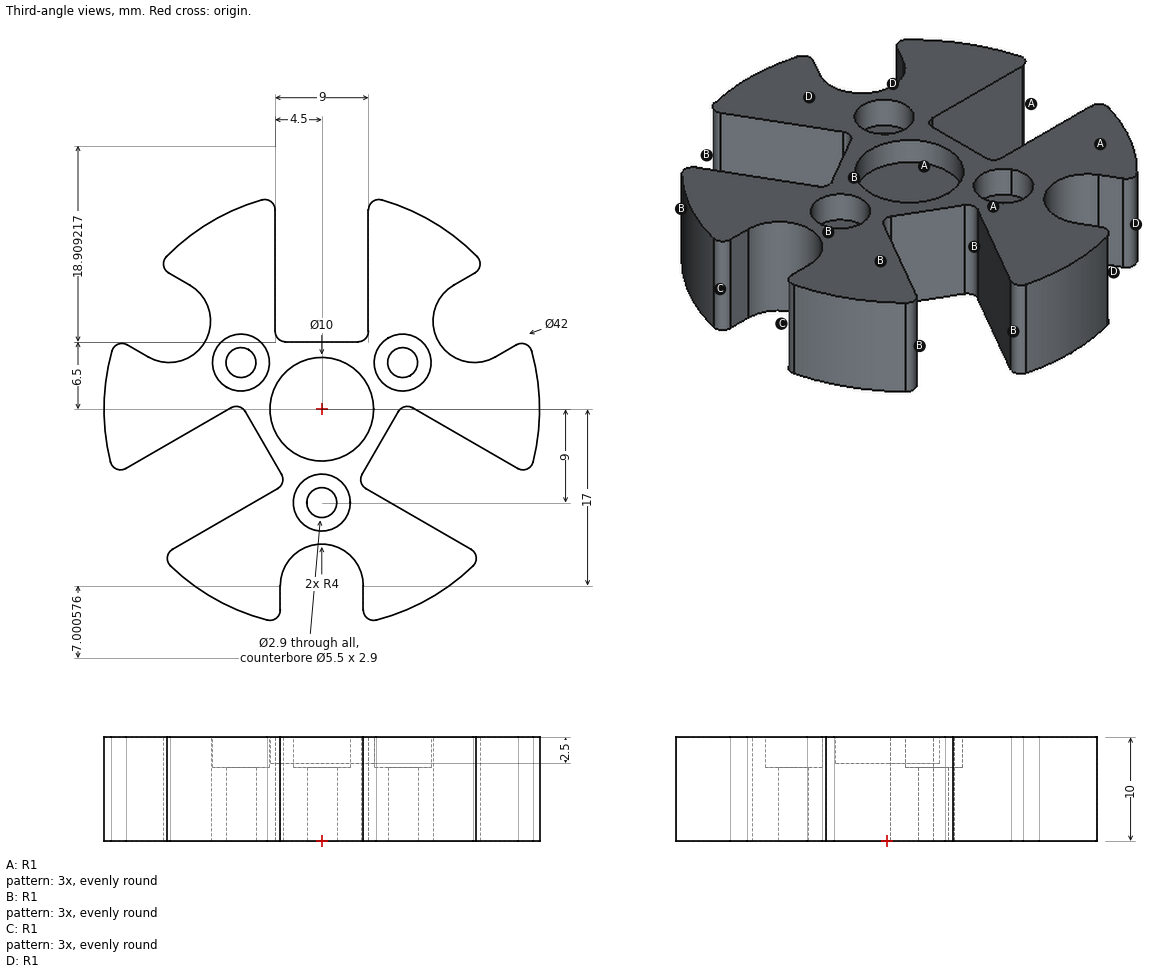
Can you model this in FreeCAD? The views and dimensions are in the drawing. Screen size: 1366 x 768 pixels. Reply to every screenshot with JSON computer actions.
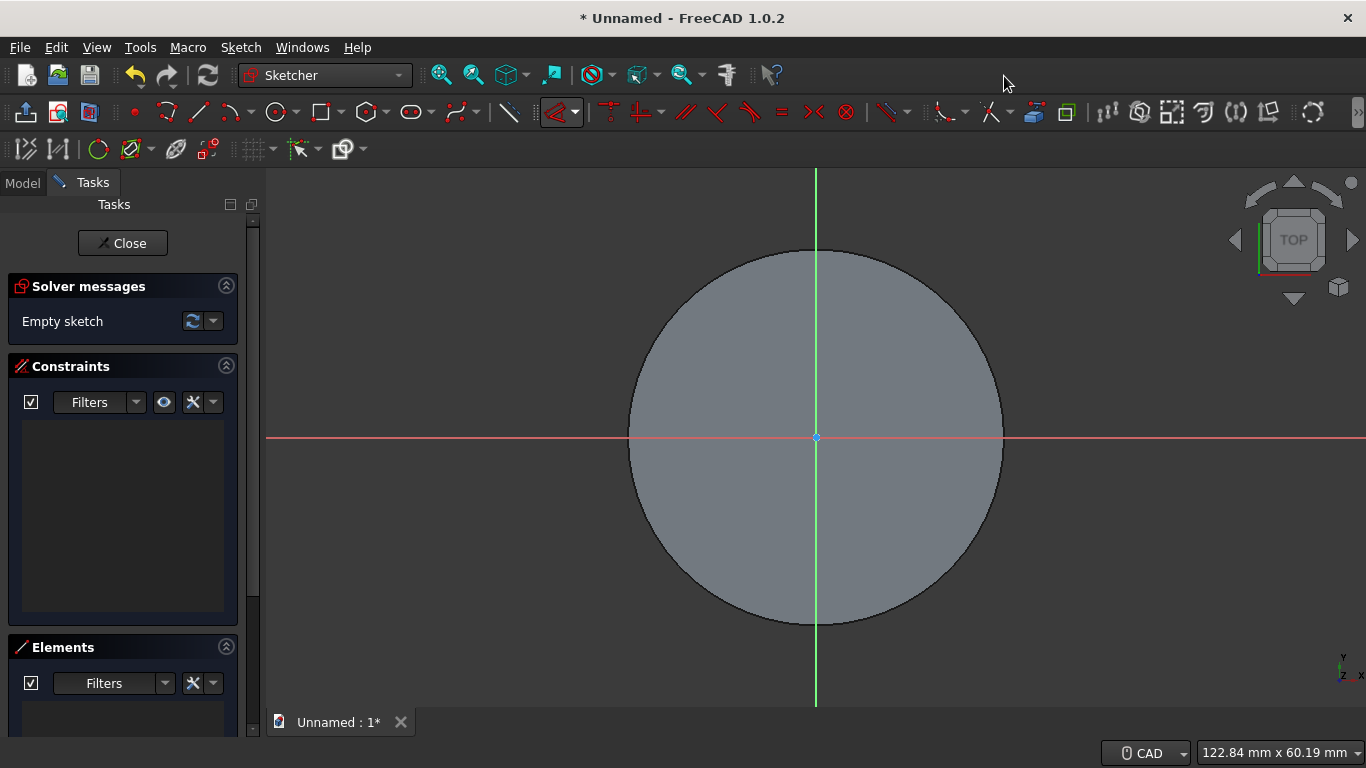
{"action": "scroll", "coordinate": [438, 679], "scroll_direction": "down", "scroll_amount": 1}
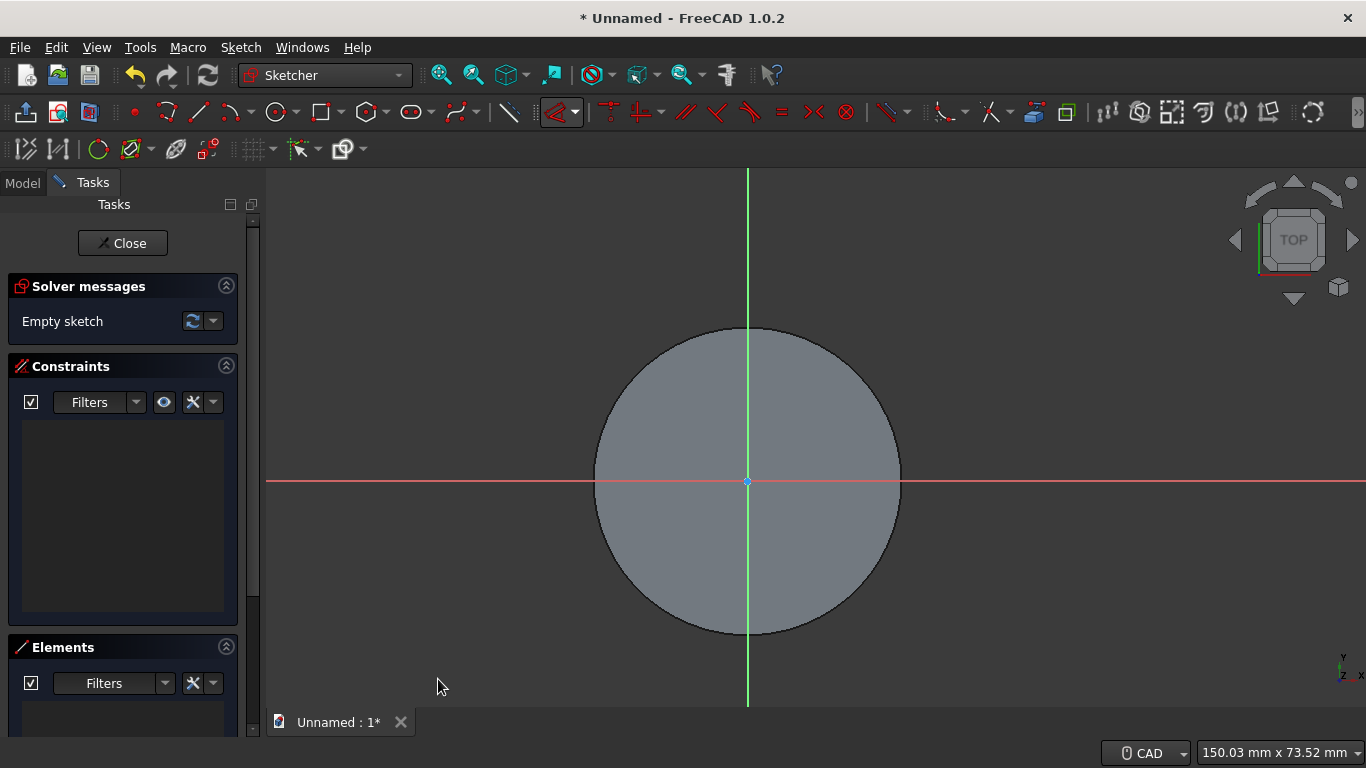
{"action": "scroll", "coordinate": [748, 328], "scroll_direction": "up", "scroll_amount": 3}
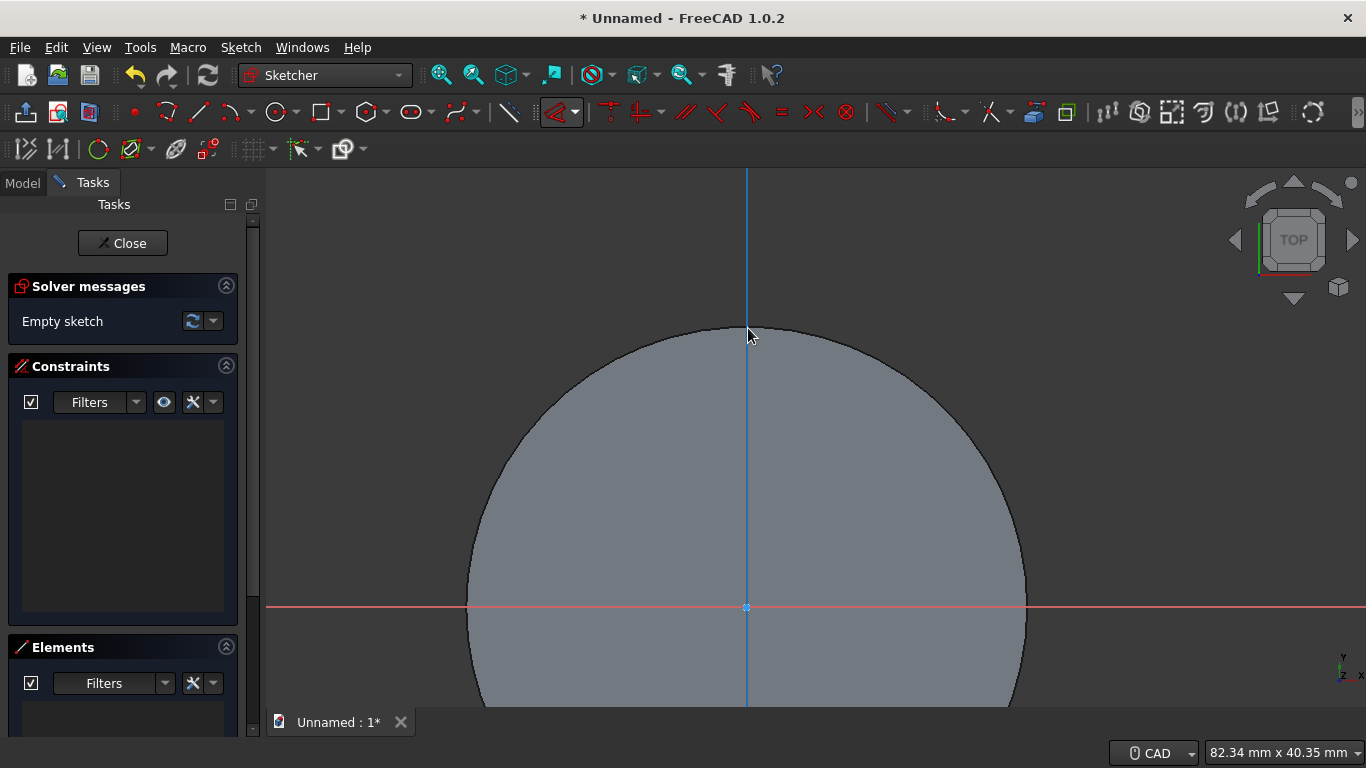
{"action": "left_click", "coordinate": [322, 112]}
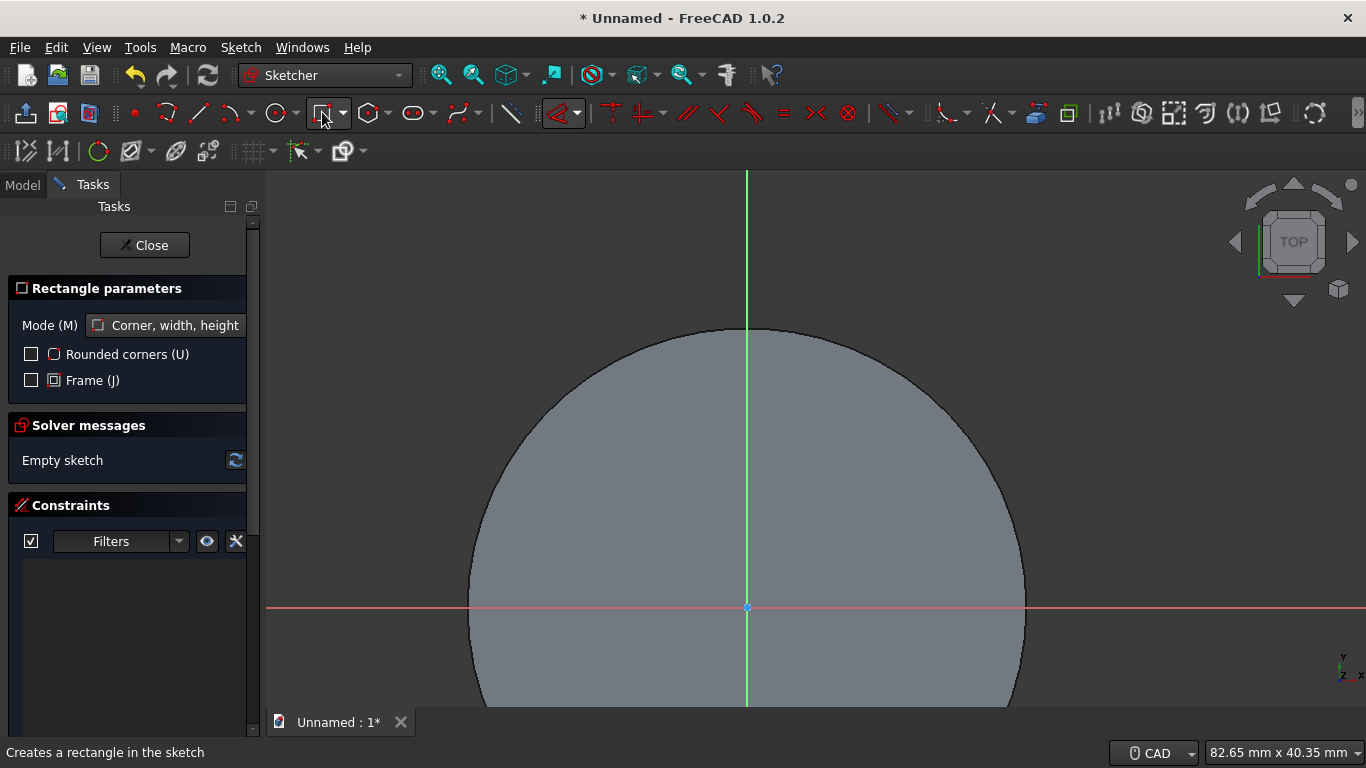
{"action": "left_click", "coordinate": [687, 270]}
{"action": "left_click", "coordinate": [807, 521]}
{"action": "key", "text": "Escape"}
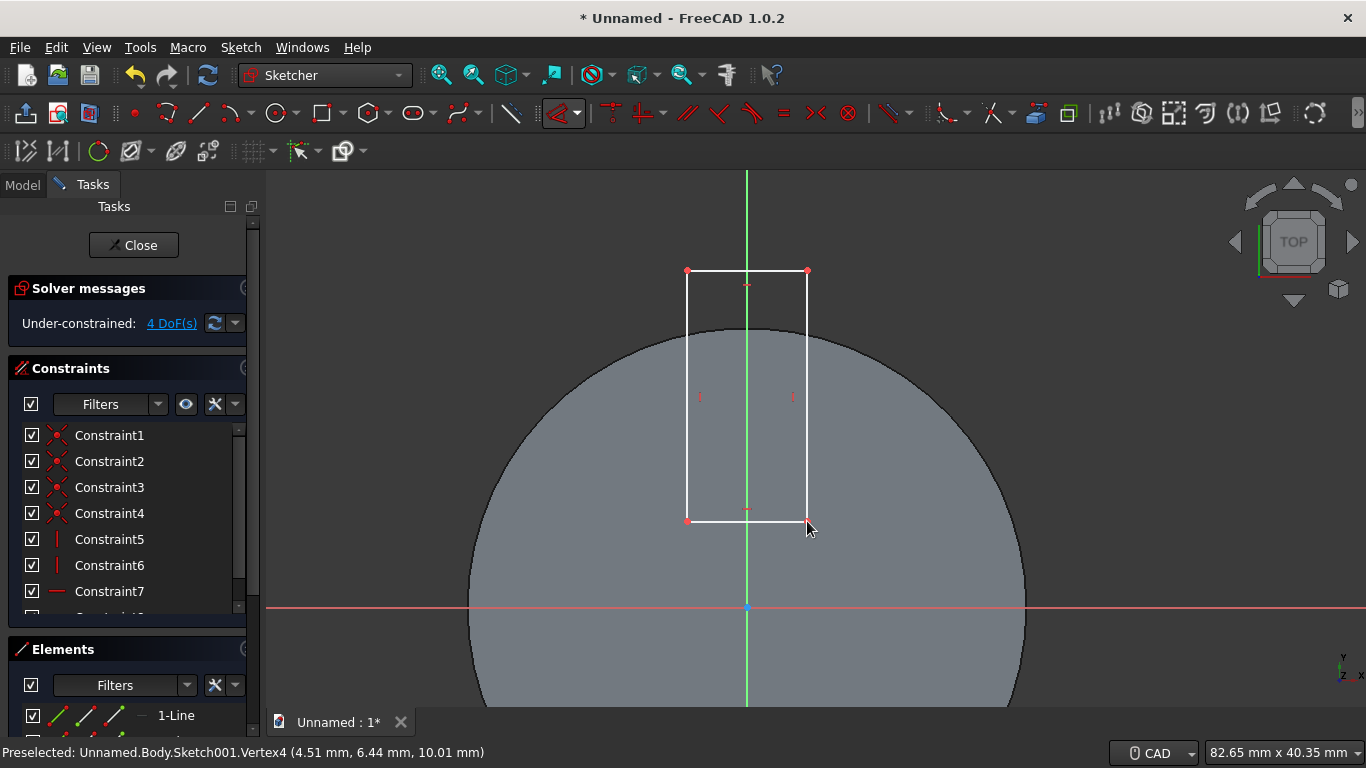
{"action": "left_click", "coordinate": [723, 522]}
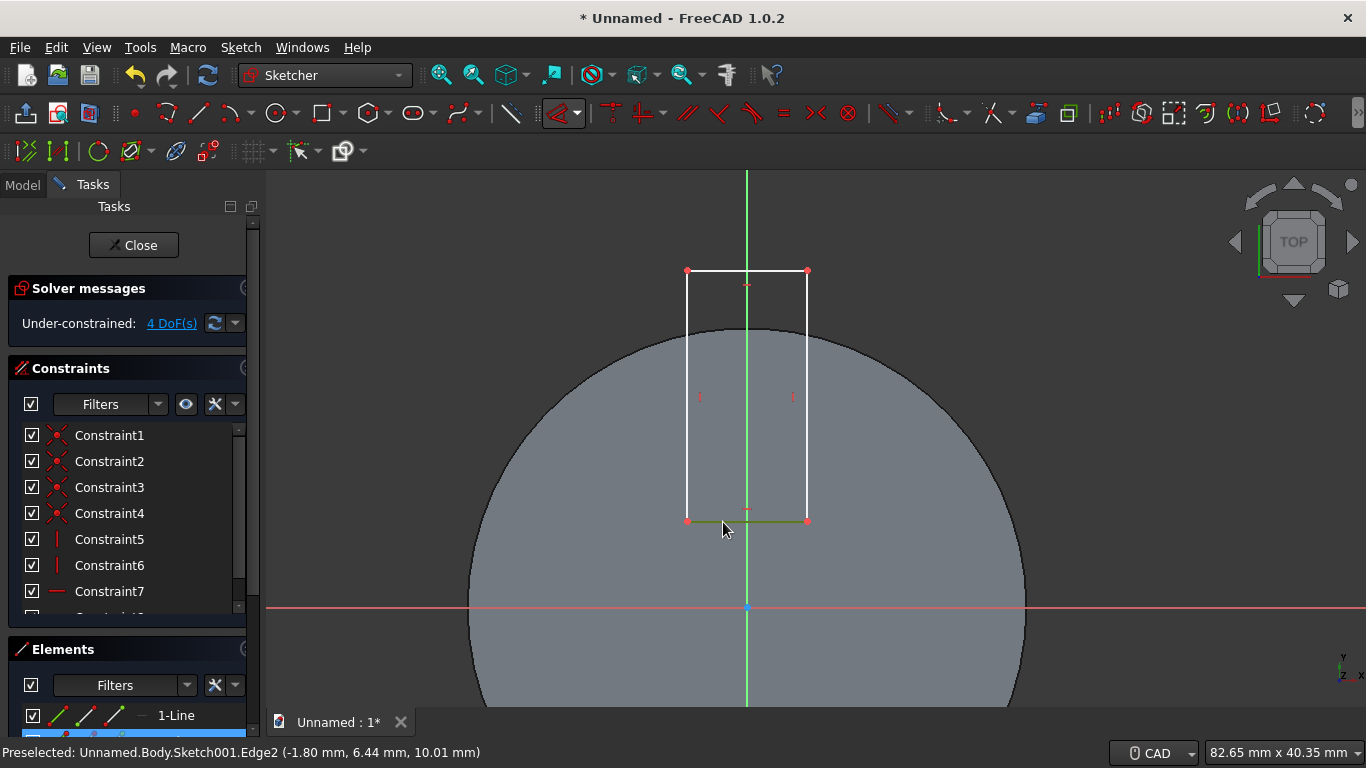
{"action": "key", "text": "l"}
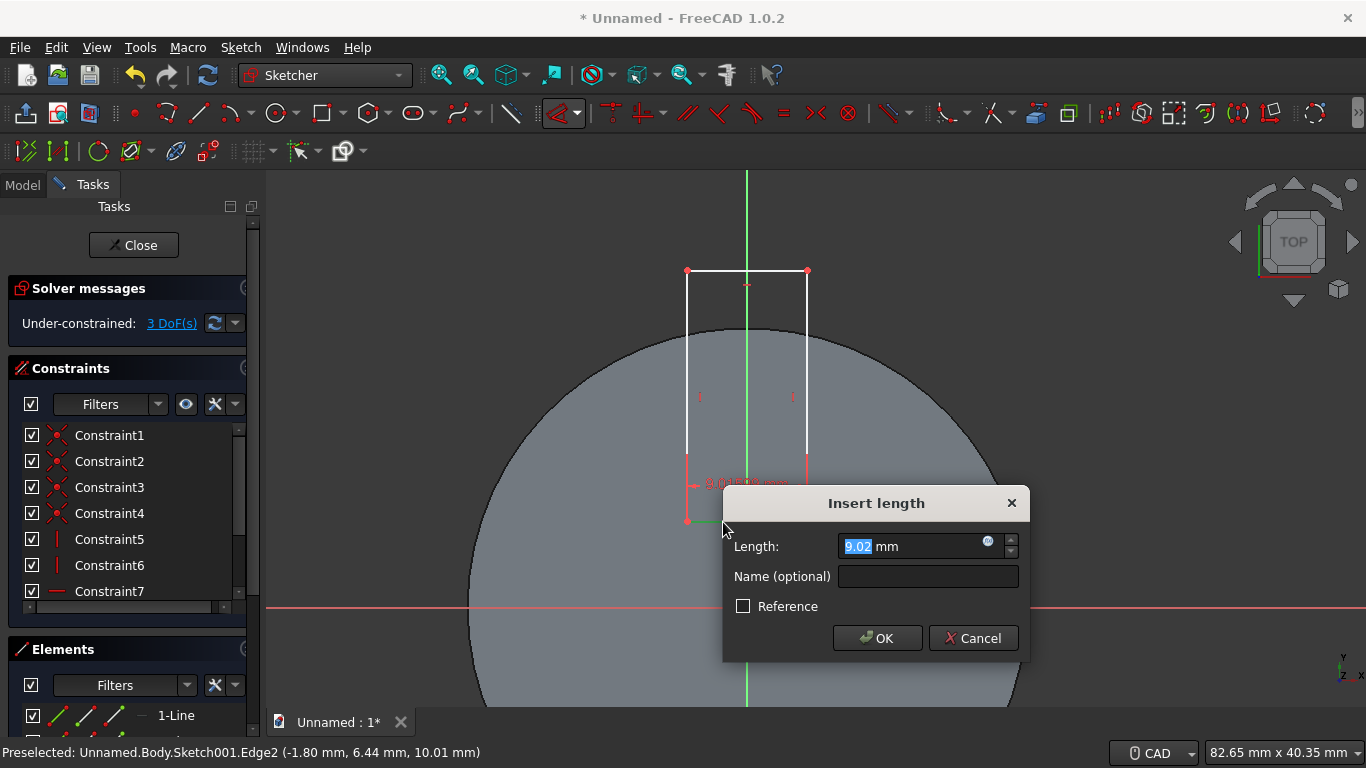
{"action": "type", "text": "9"}
{"action": "key", "text": "Return"}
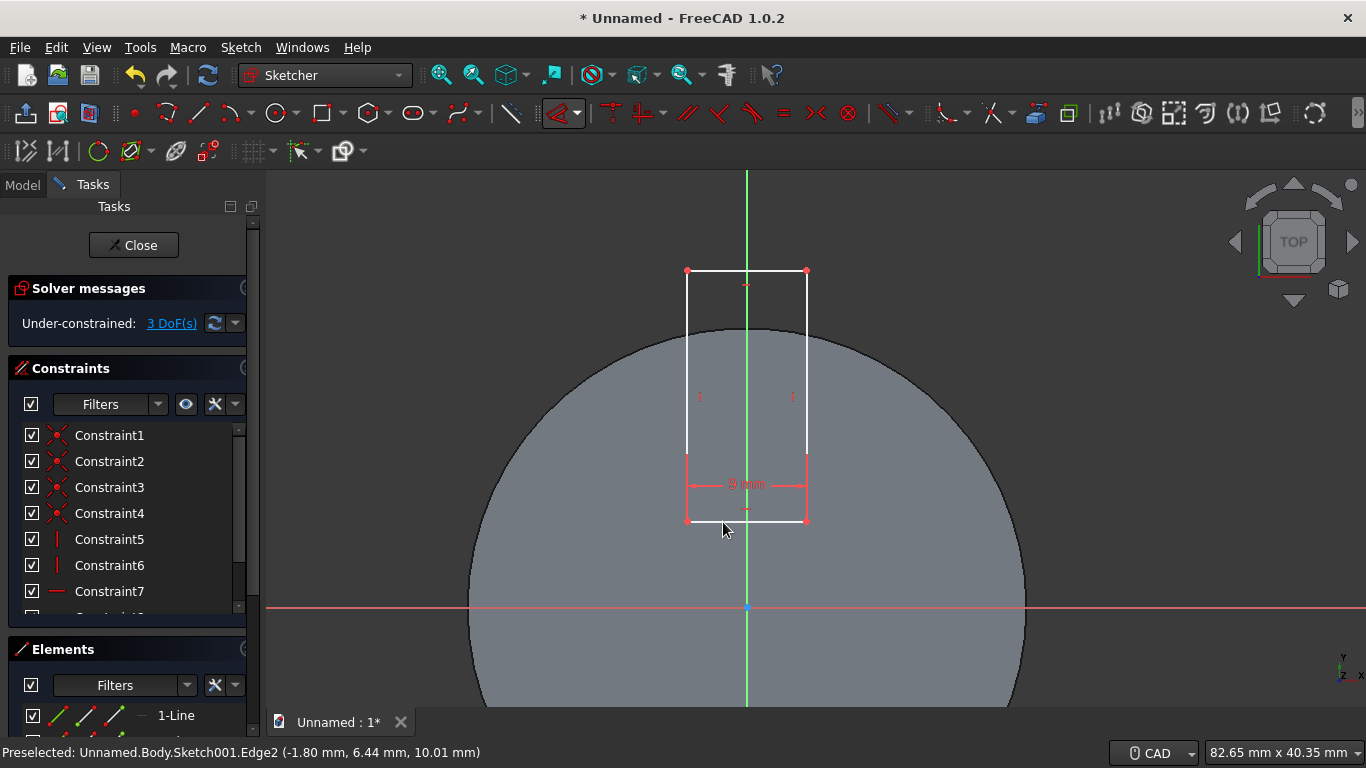
{"action": "left_click", "coordinate": [687, 271]}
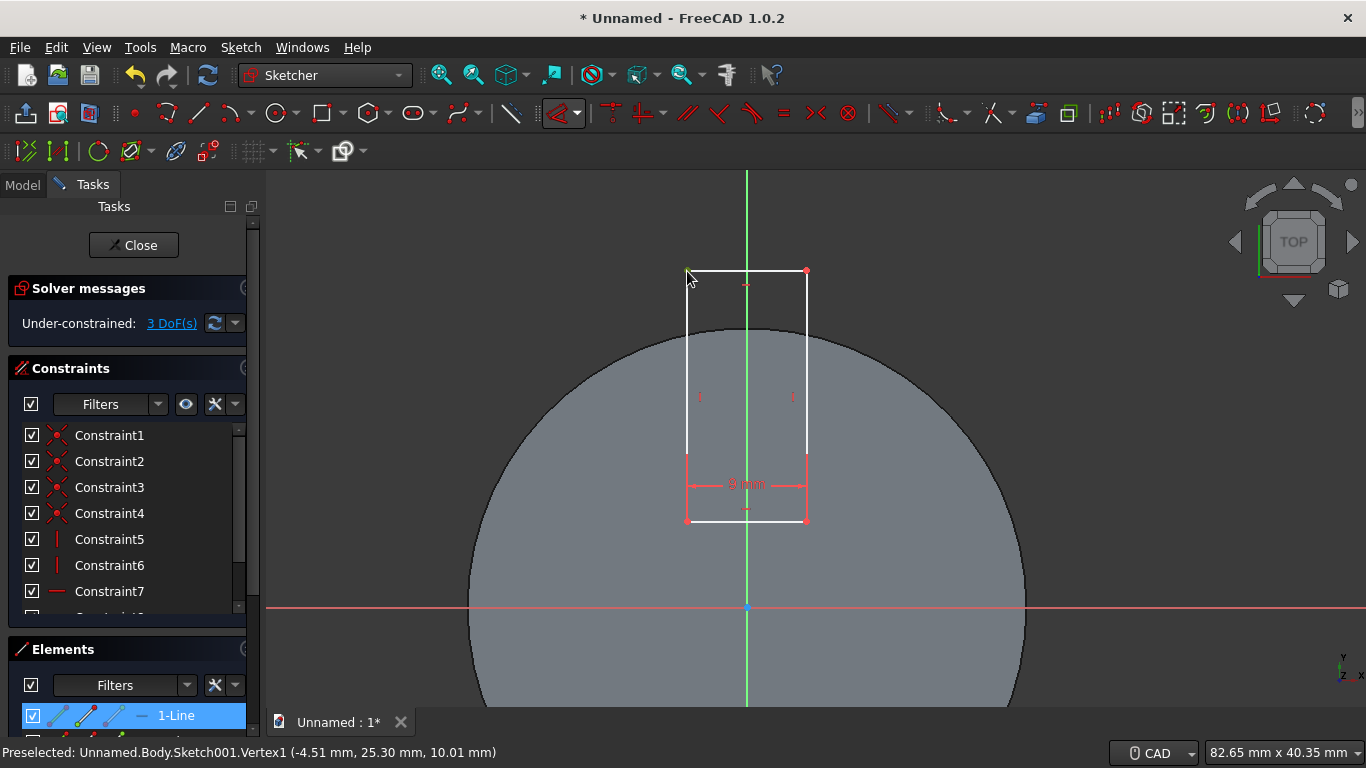
{"action": "left_click", "coordinate": [580, 114]}